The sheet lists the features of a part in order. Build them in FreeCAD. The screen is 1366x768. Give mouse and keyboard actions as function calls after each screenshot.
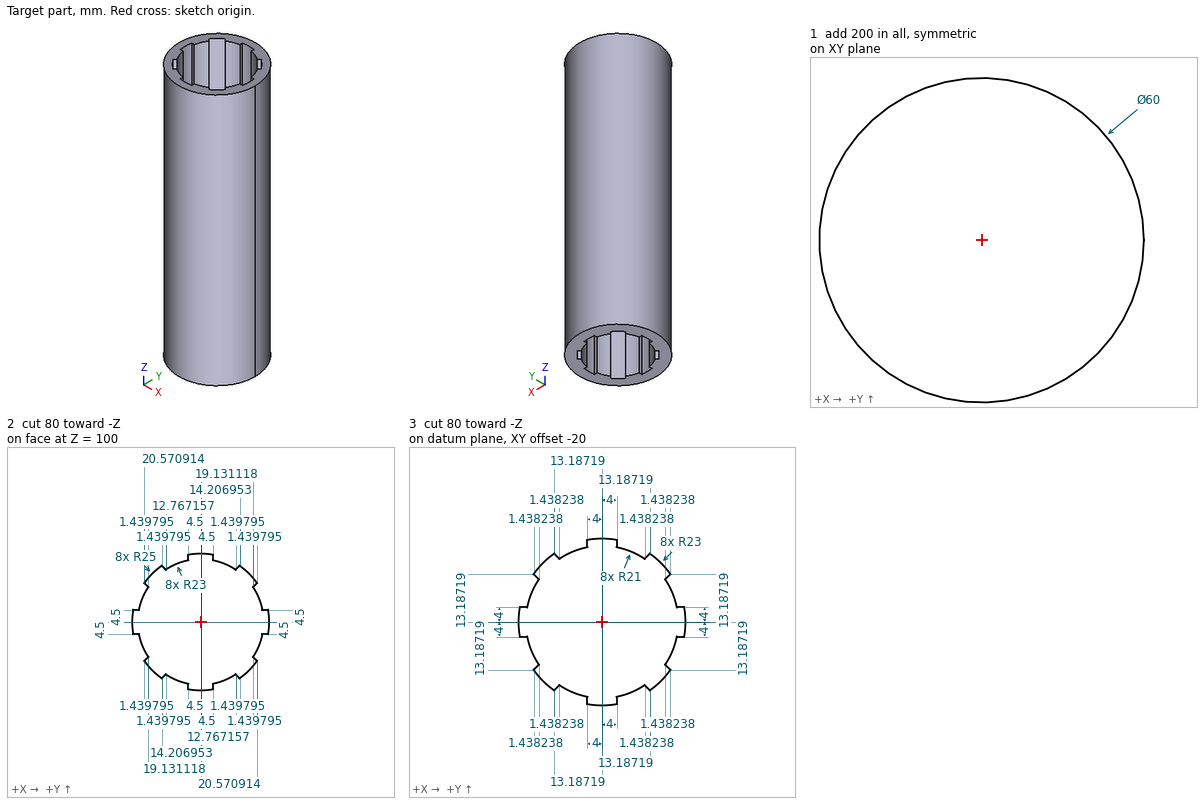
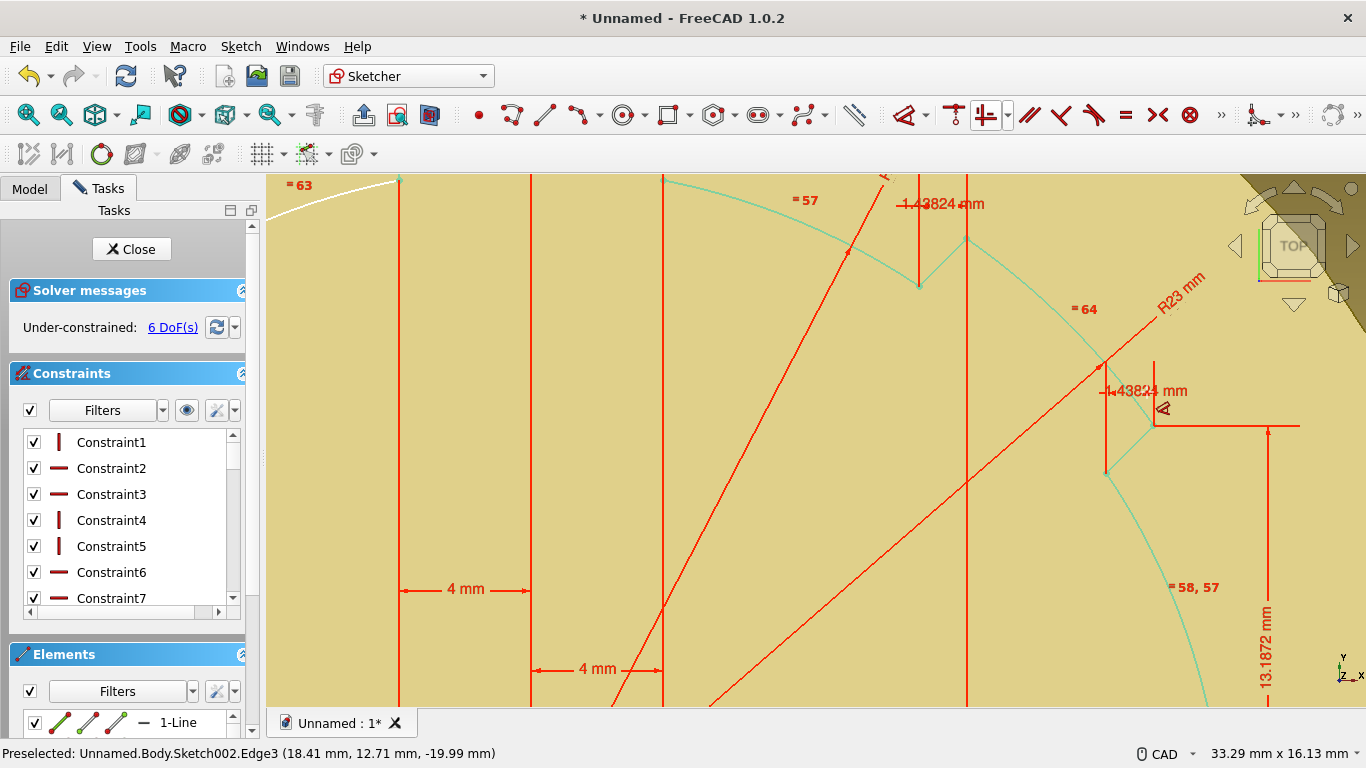
scroll(802, 334, down, 8)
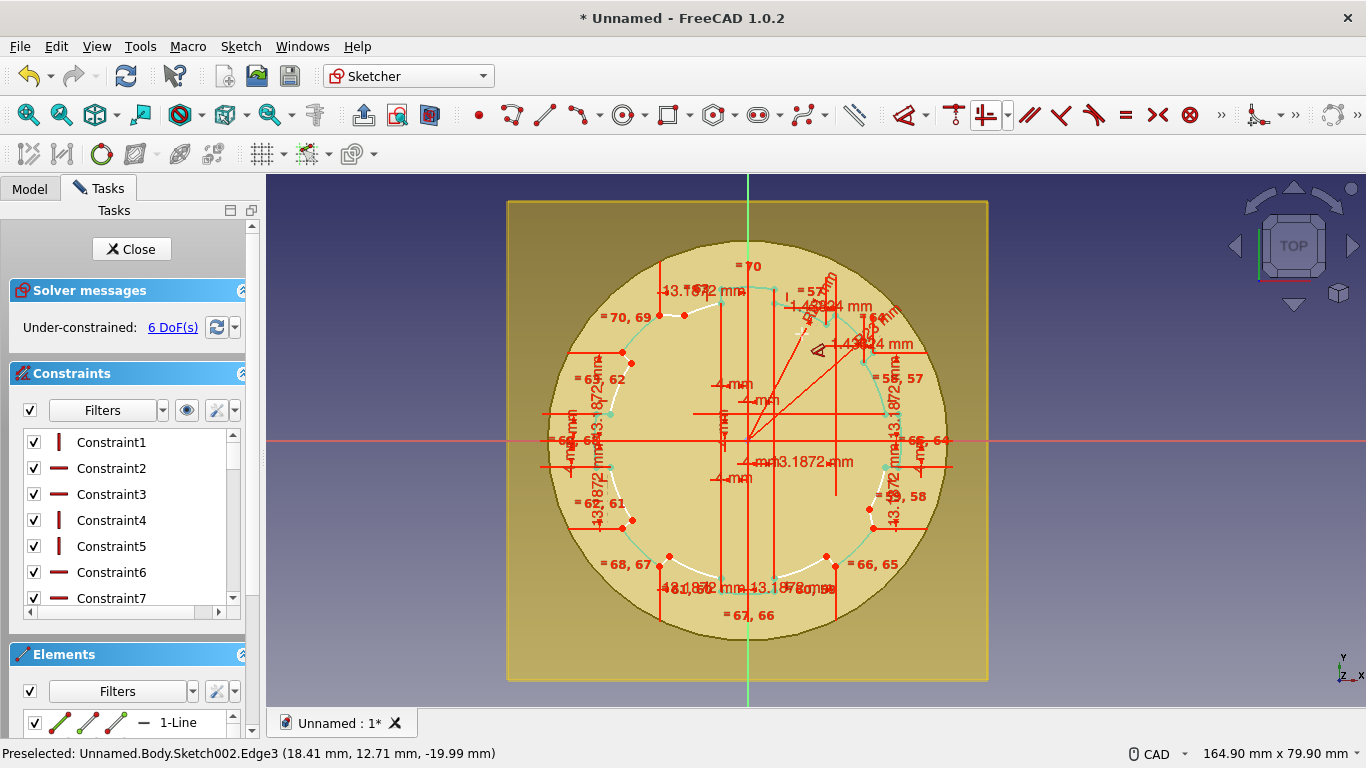
scroll(871, 516, up, 8)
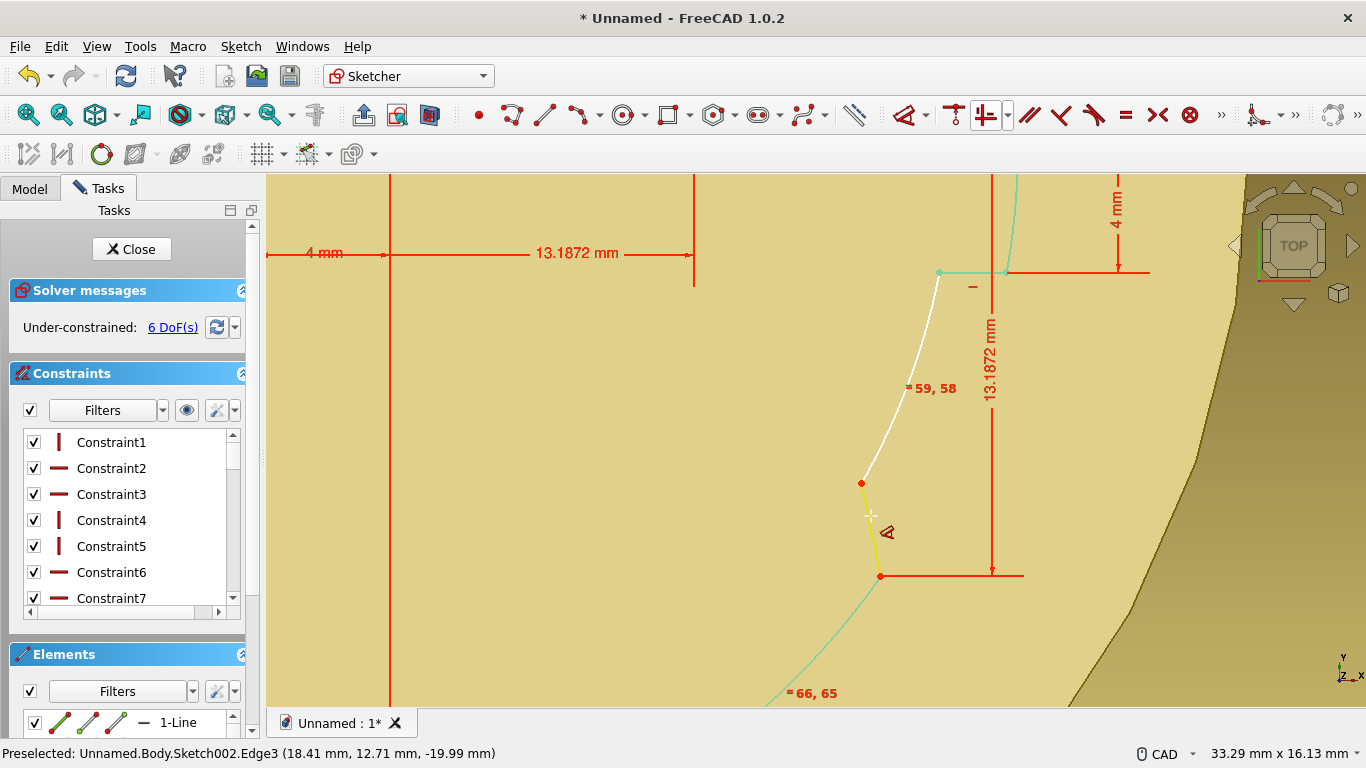
click(867, 512)
click(876, 610)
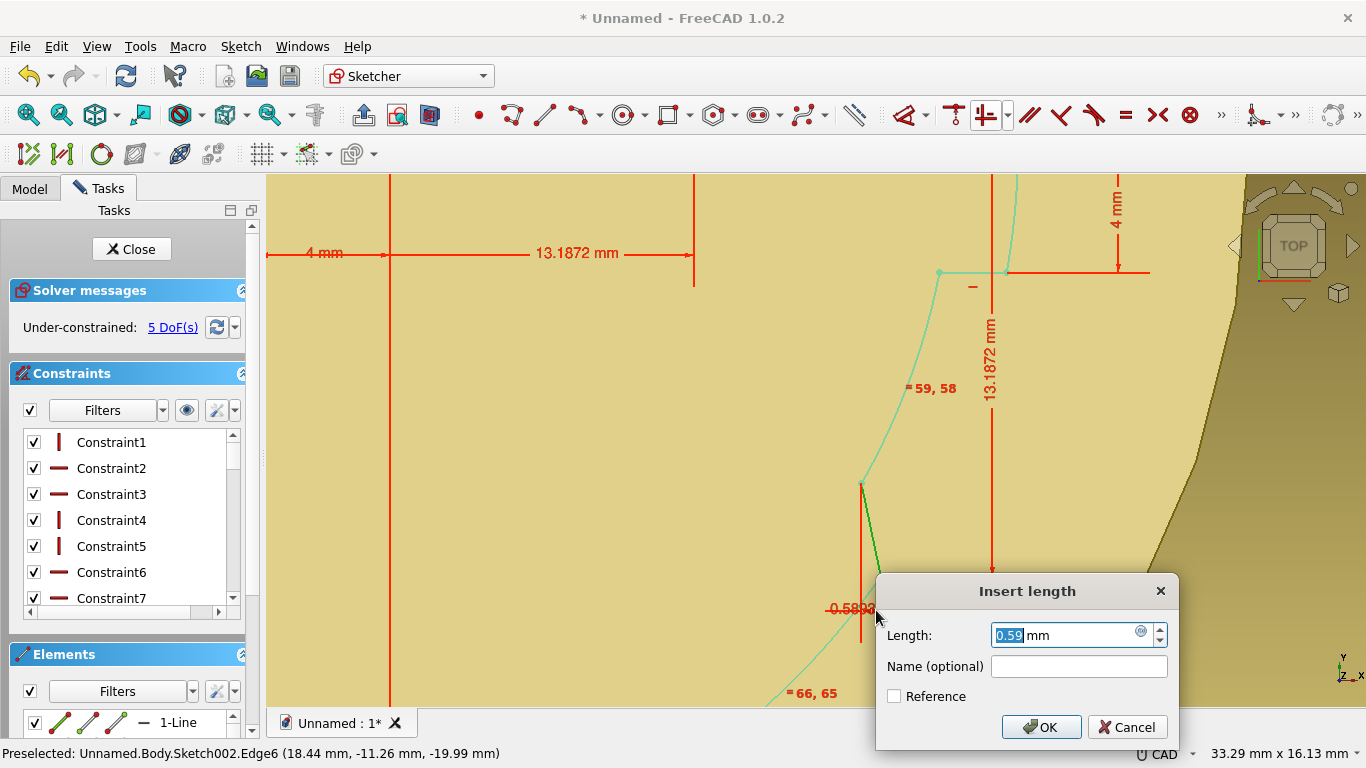
text(1.438238)
key(Return)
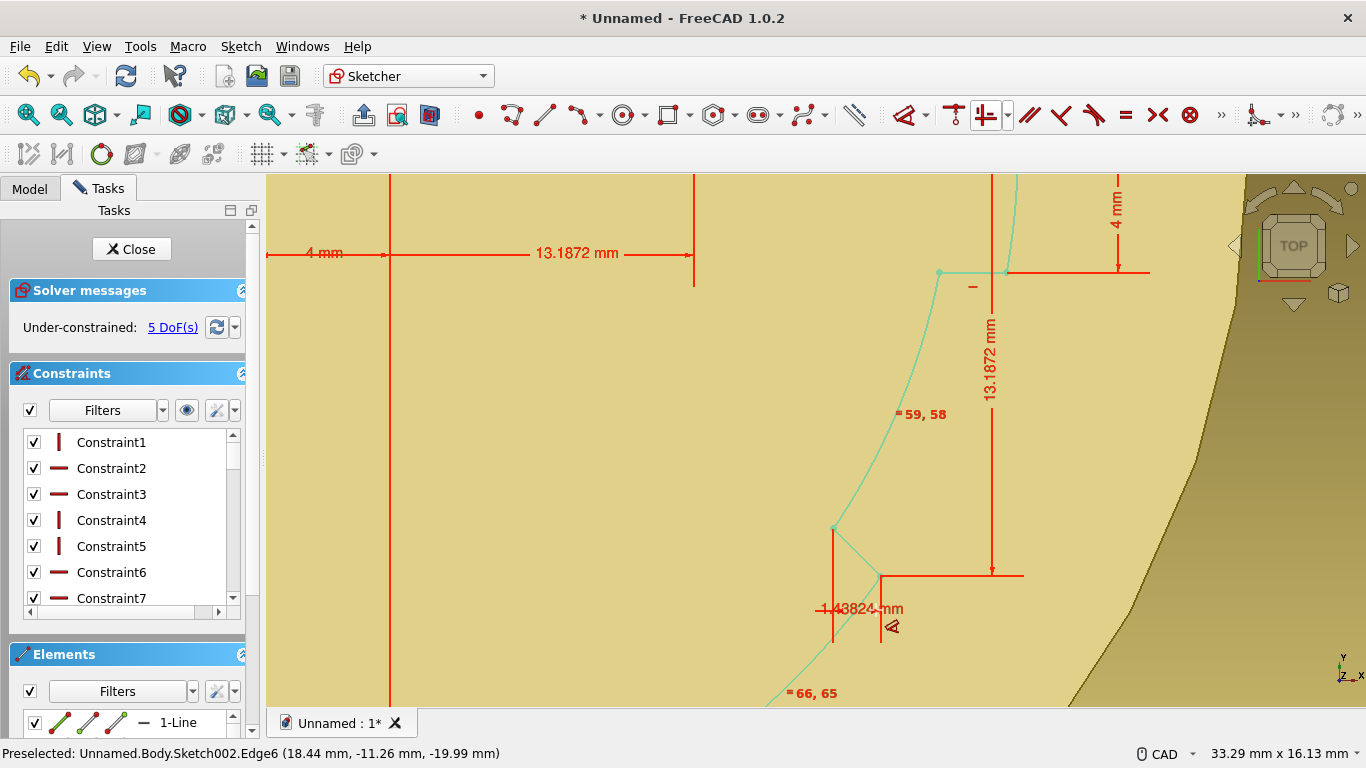
scroll(871, 516, down, 8)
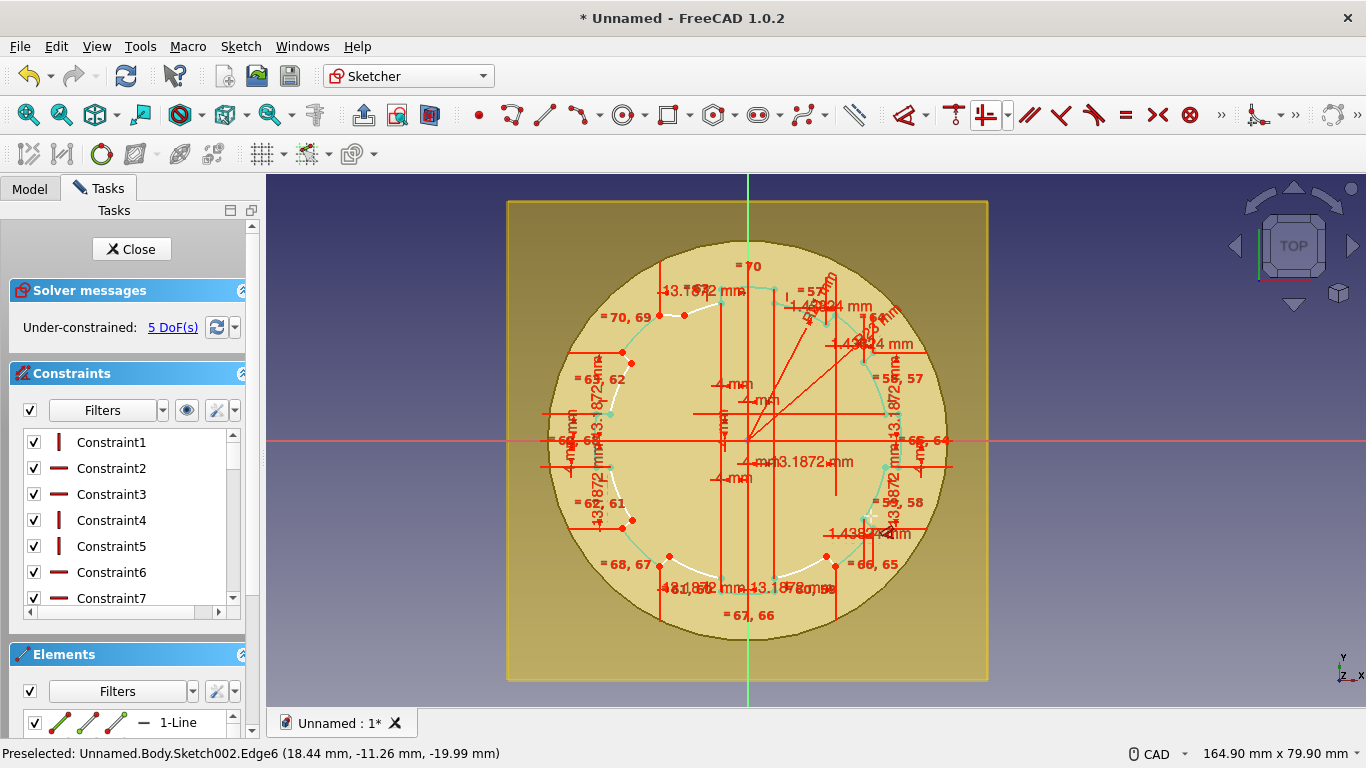
scroll(833, 563, up, 8)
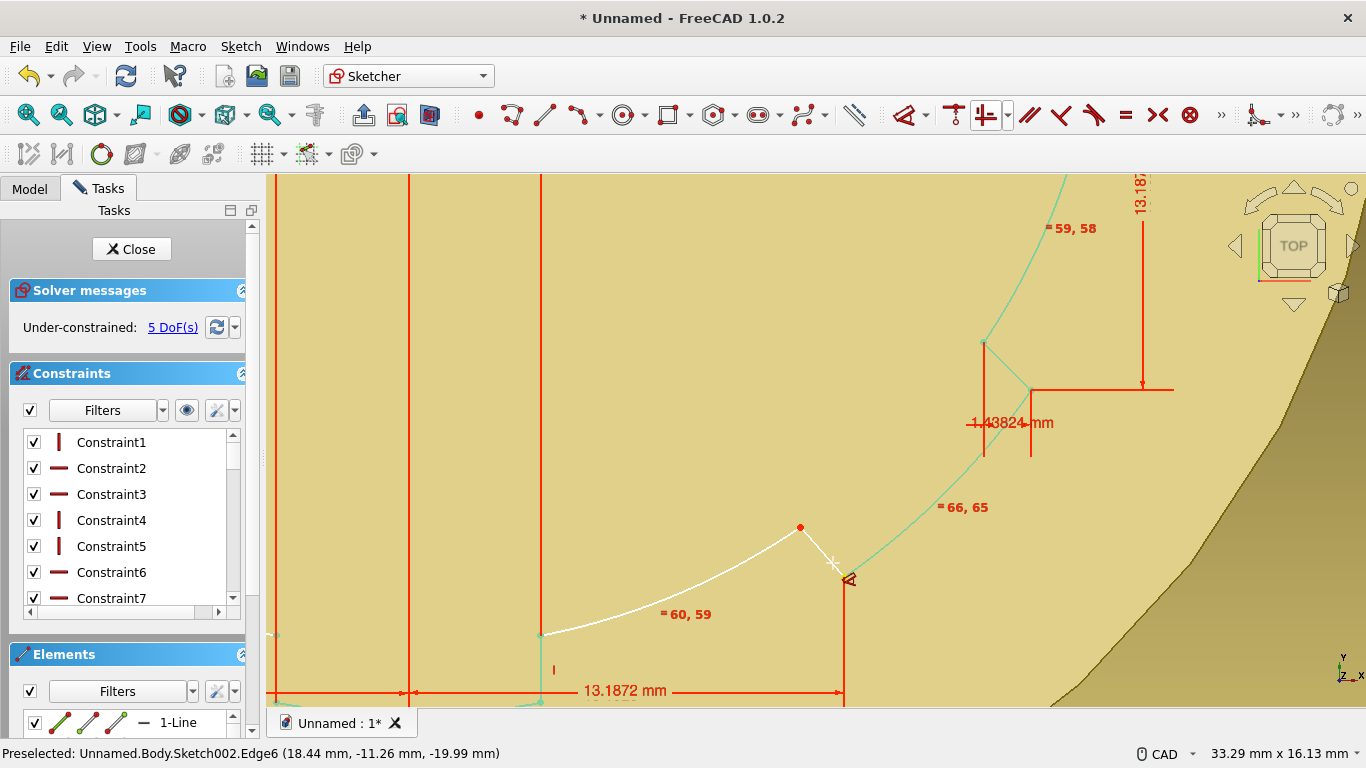
click(831, 562)
click(822, 611)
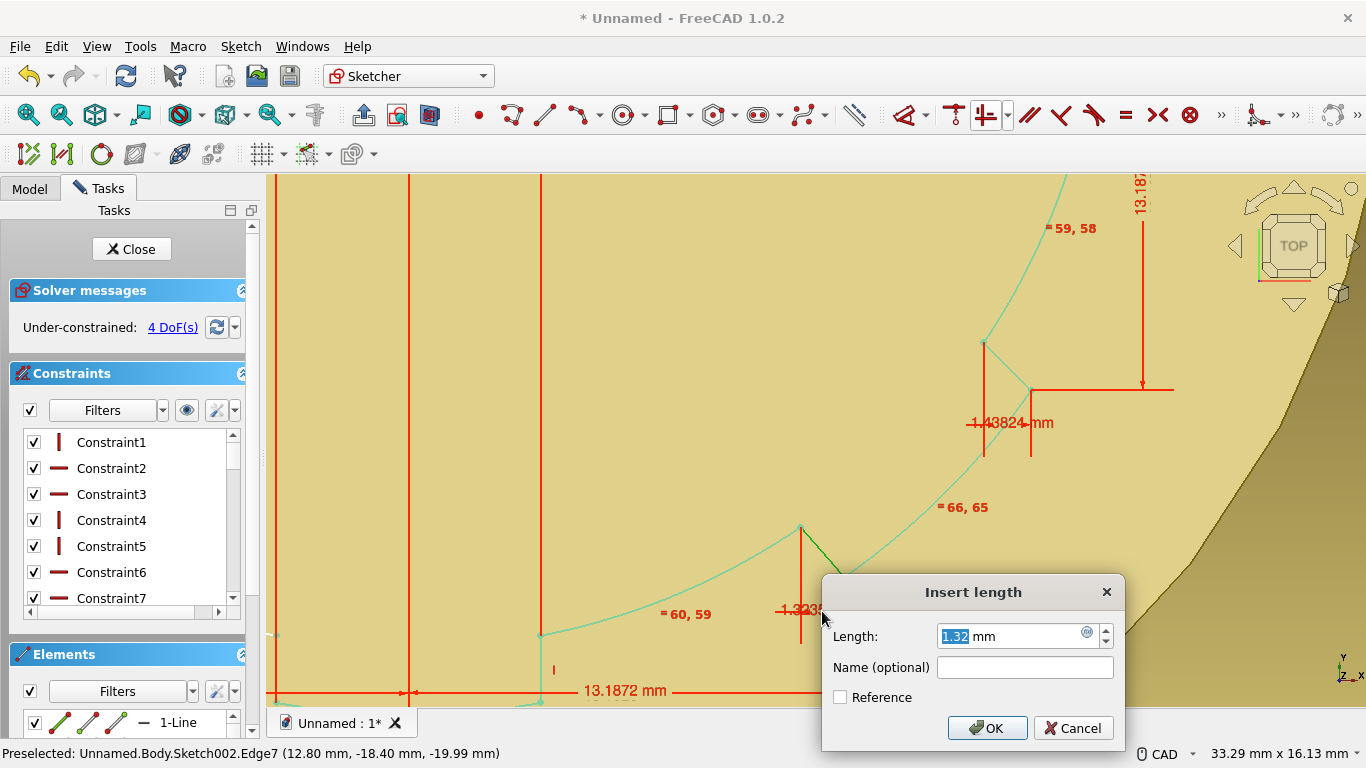
text(1.438238)
key(Return)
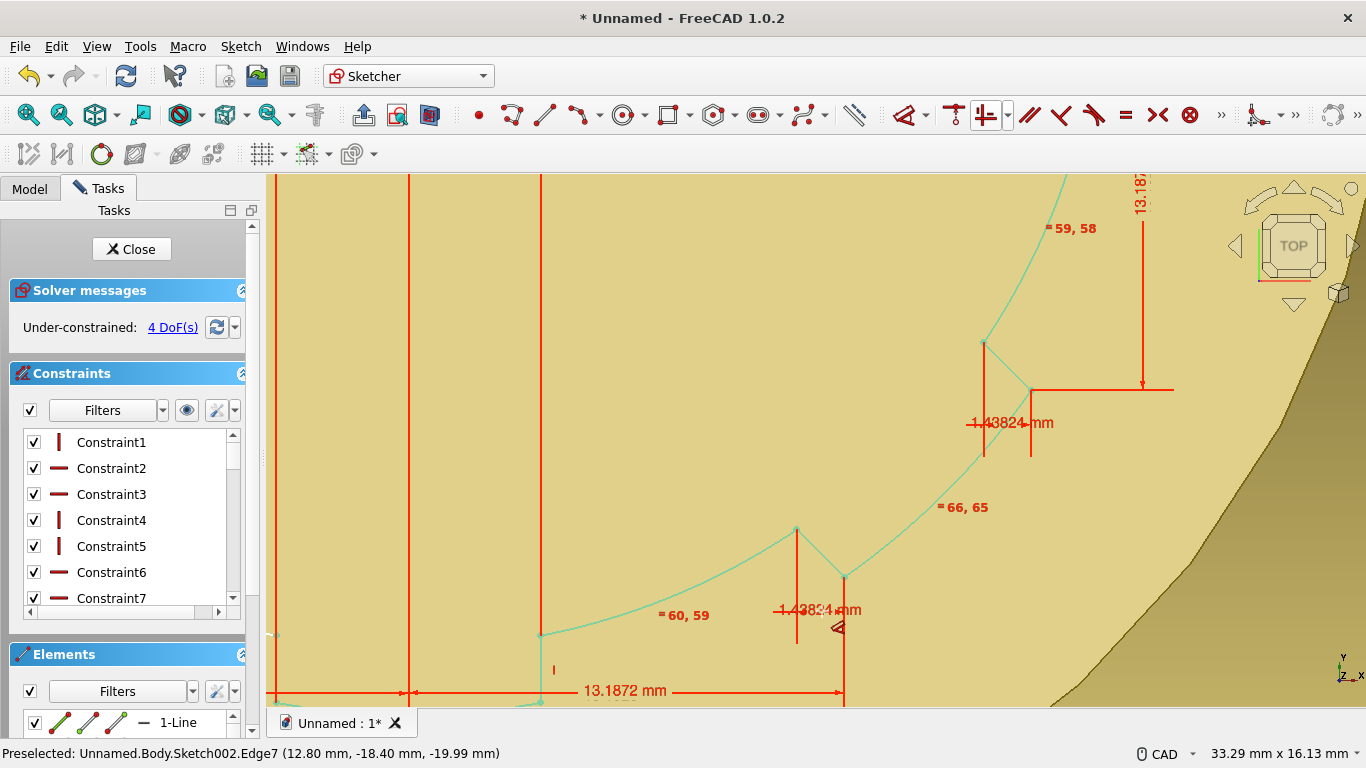
scroll(833, 563, down, 8)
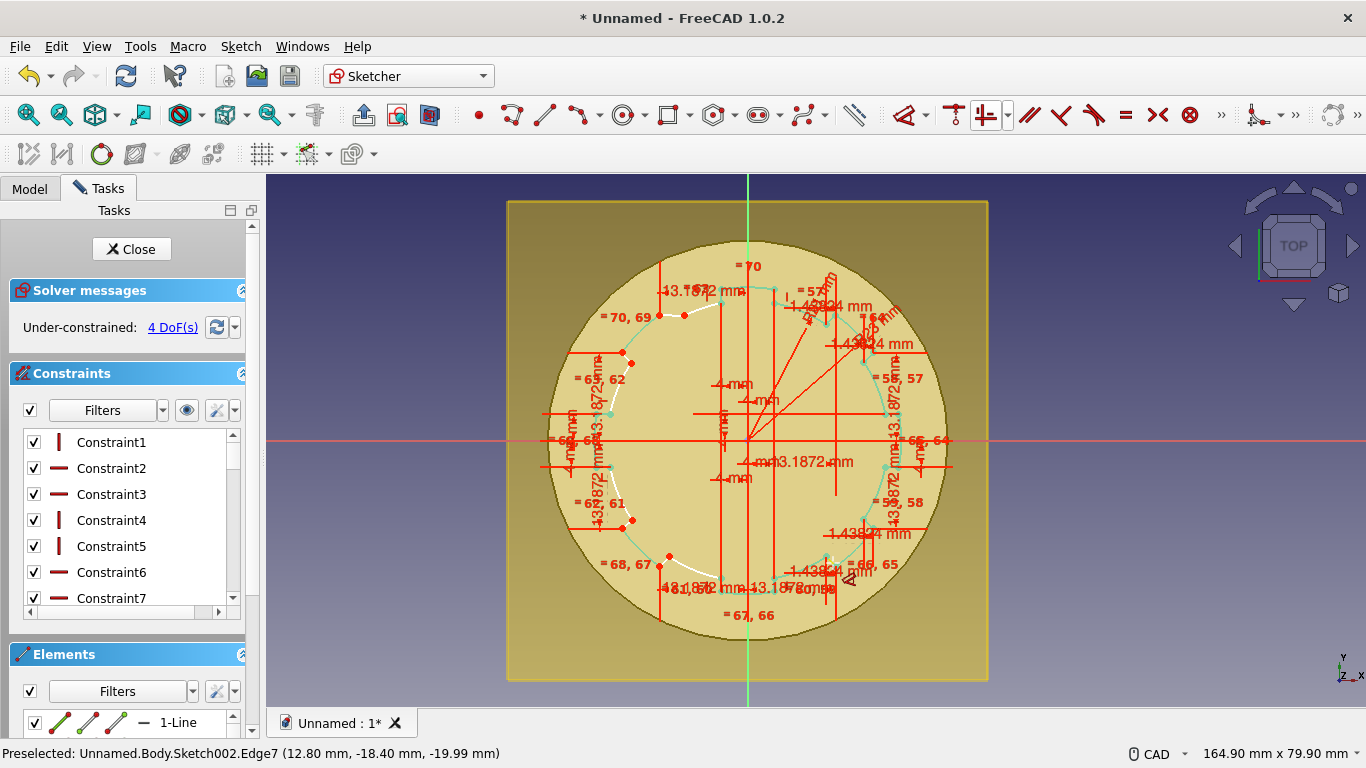
scroll(666, 560, up, 8)